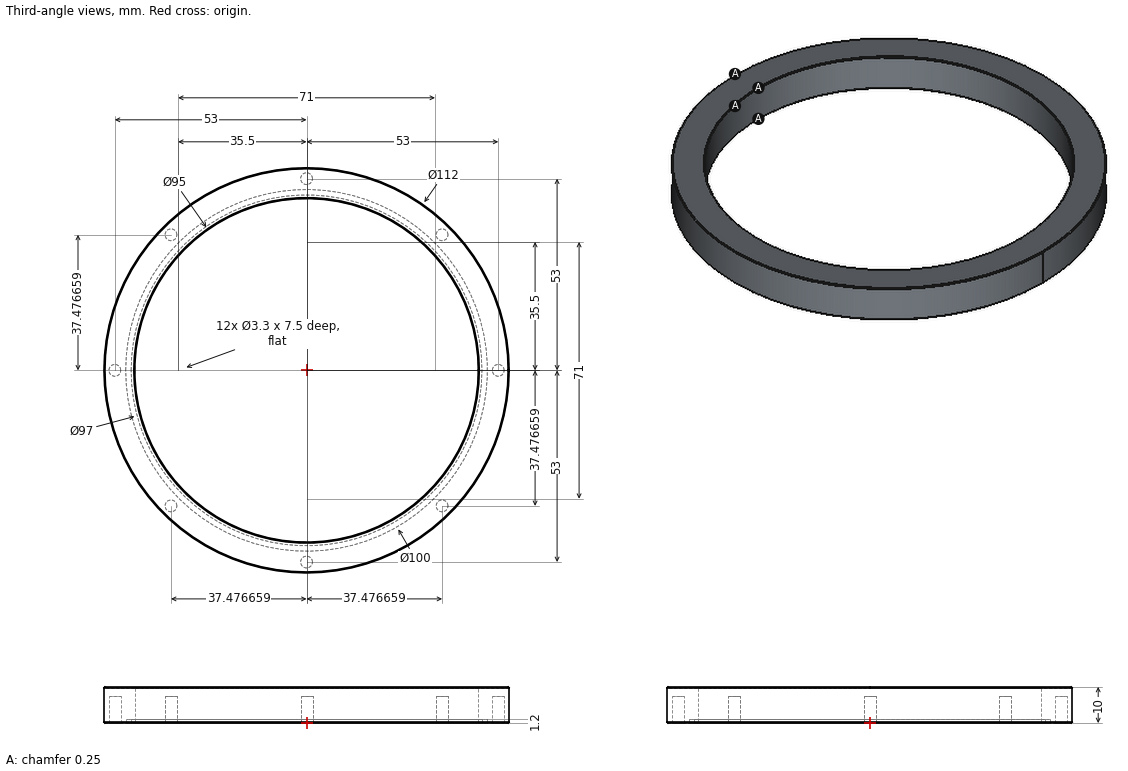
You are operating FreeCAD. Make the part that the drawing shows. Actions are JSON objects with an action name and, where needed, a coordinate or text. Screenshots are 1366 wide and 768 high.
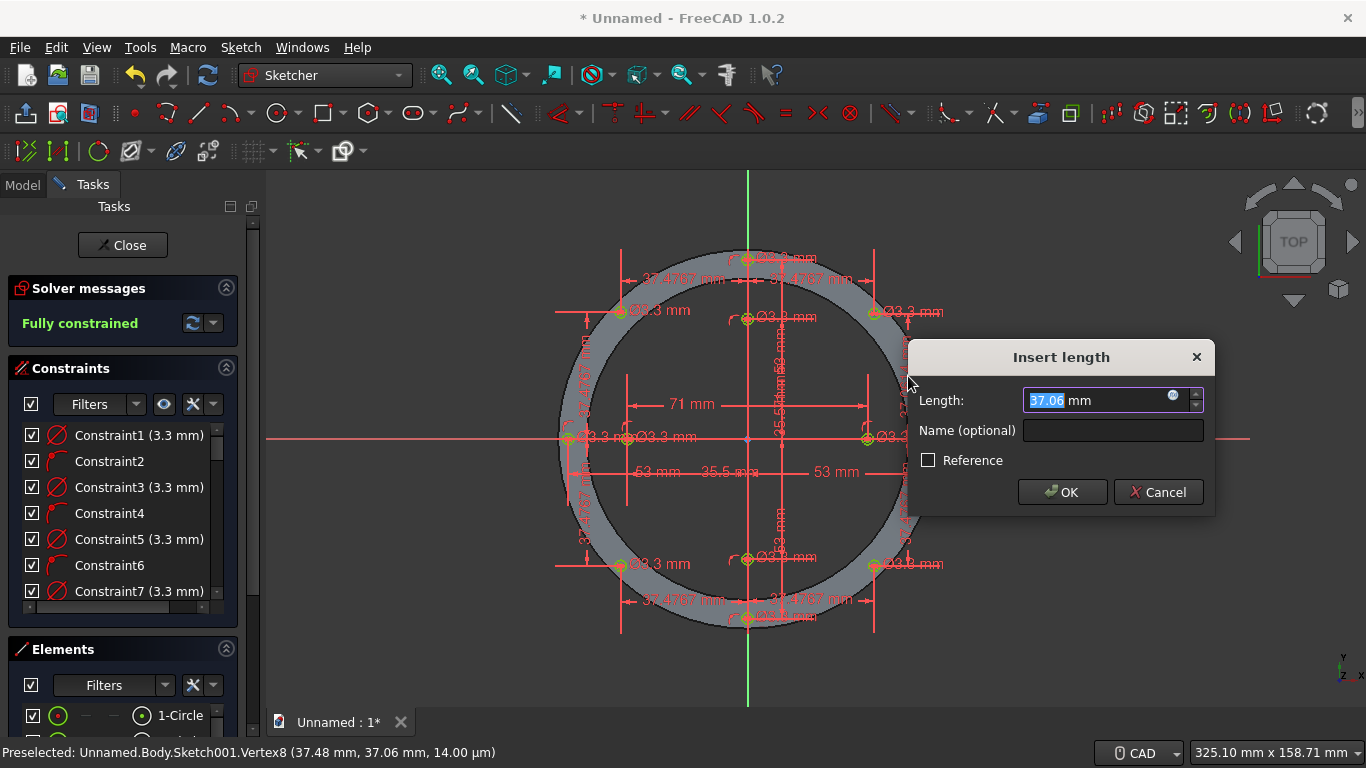
{"action": "type", "text": "37.476659"}
{"action": "key", "text": "Return"}
{"action": "key", "text": "Escape"}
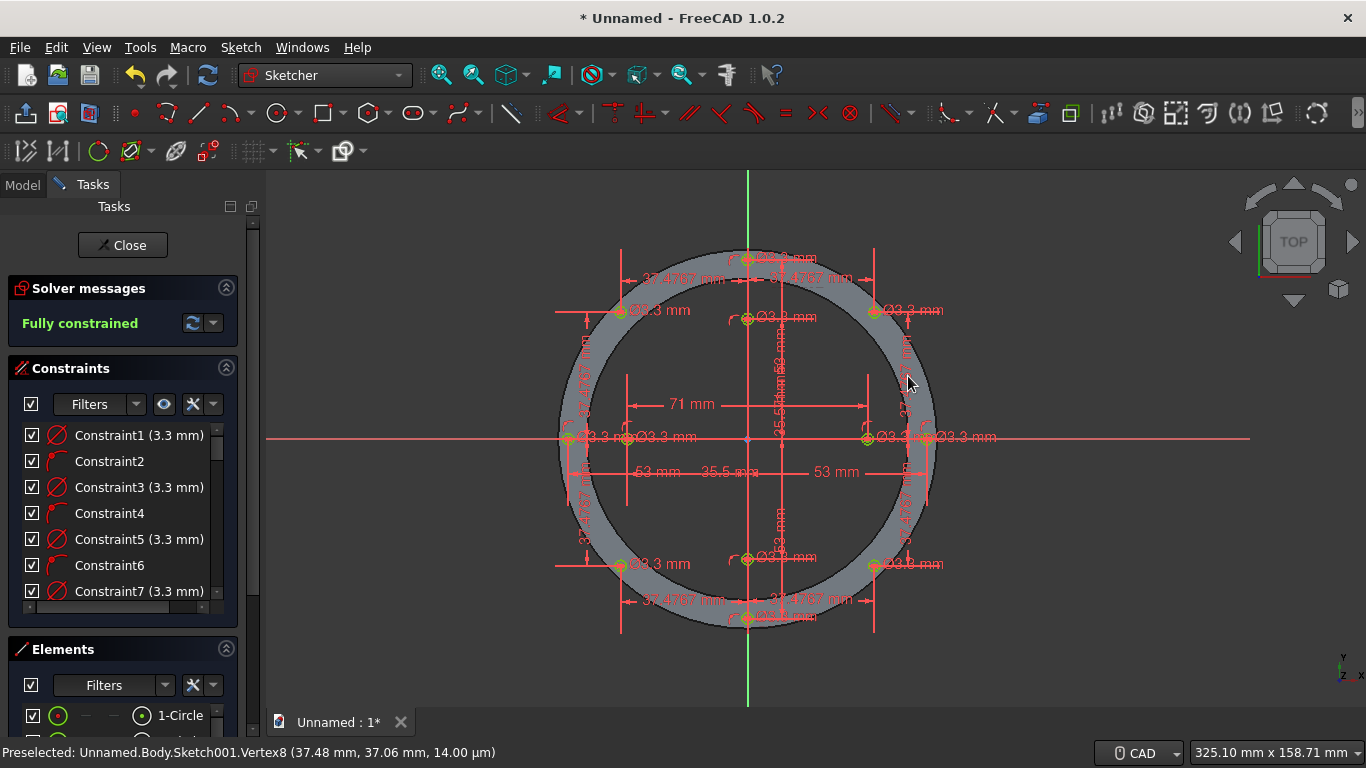
{"action": "left_click", "coordinate": [123, 245]}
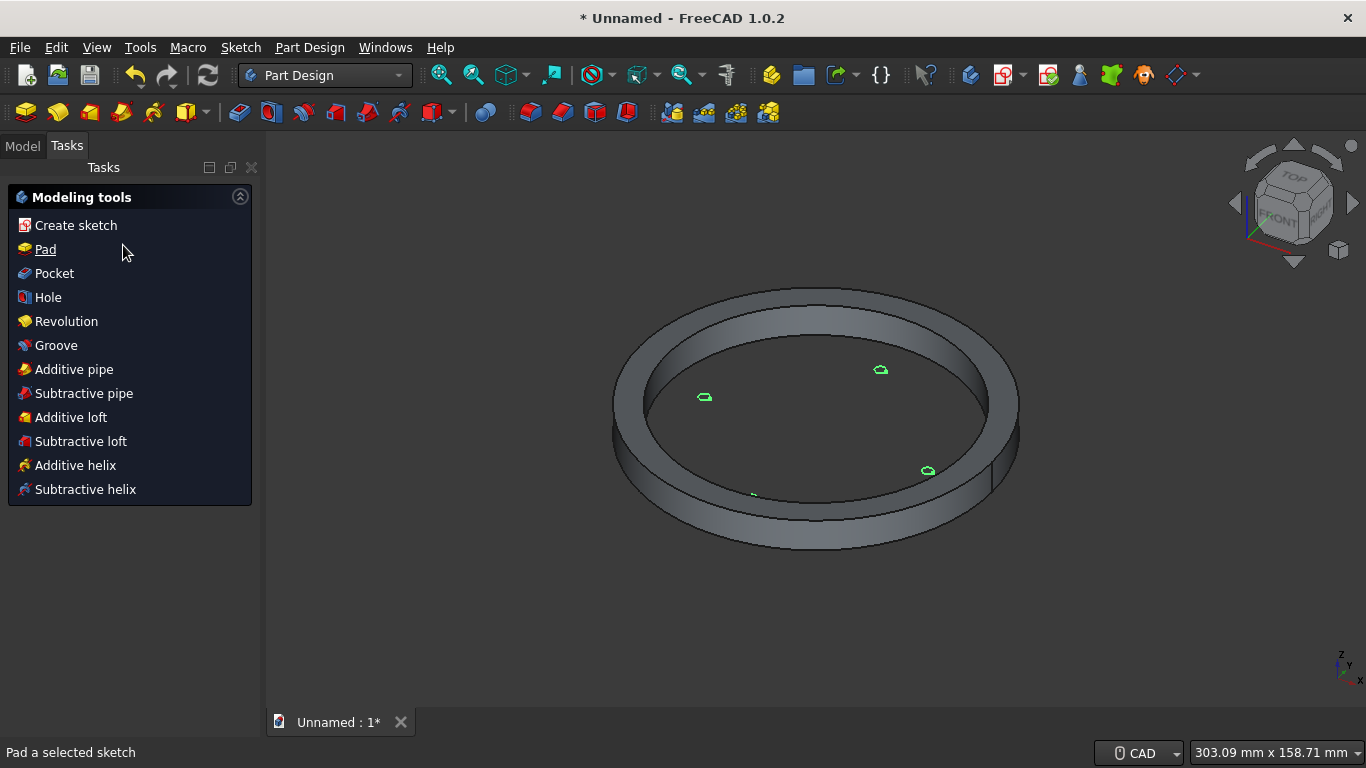
{"action": "left_click", "coordinate": [272, 112]}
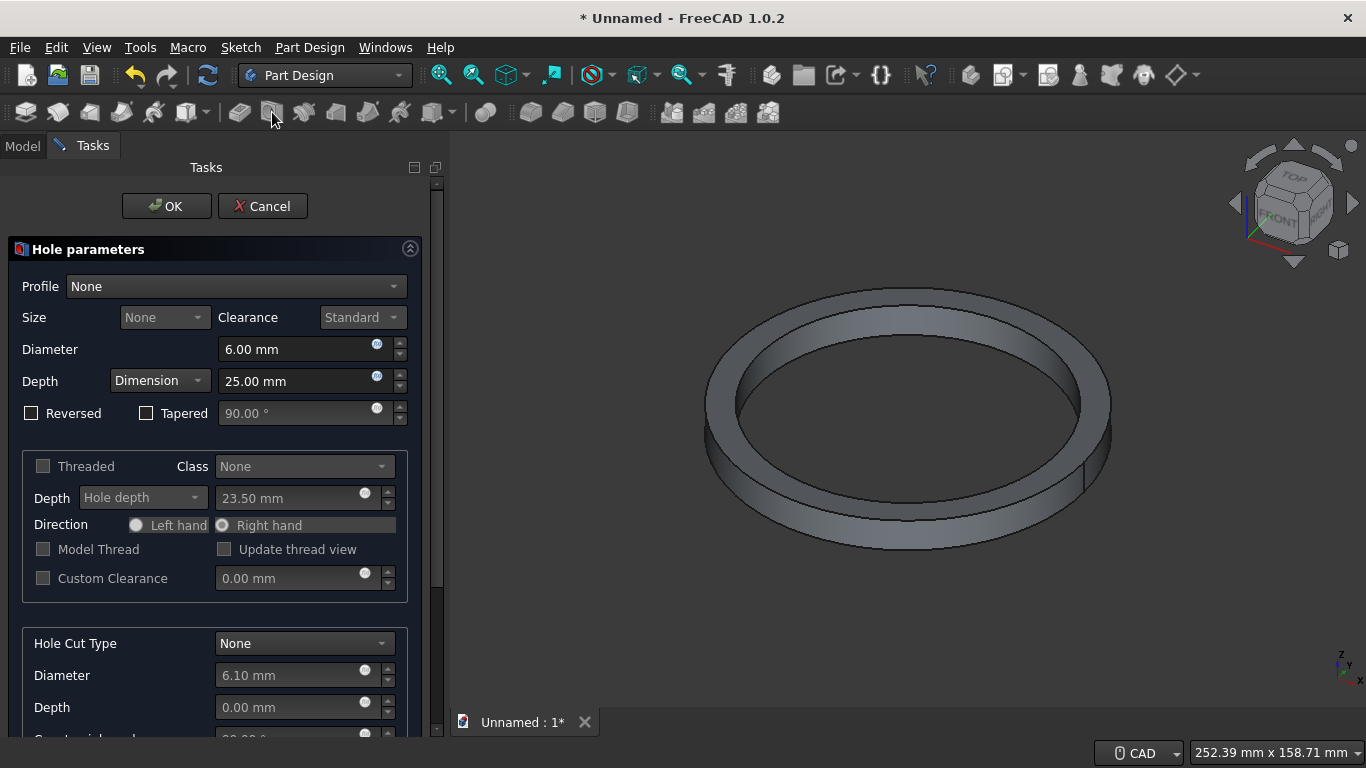
{"action": "triple_click", "coordinate": [305, 349]}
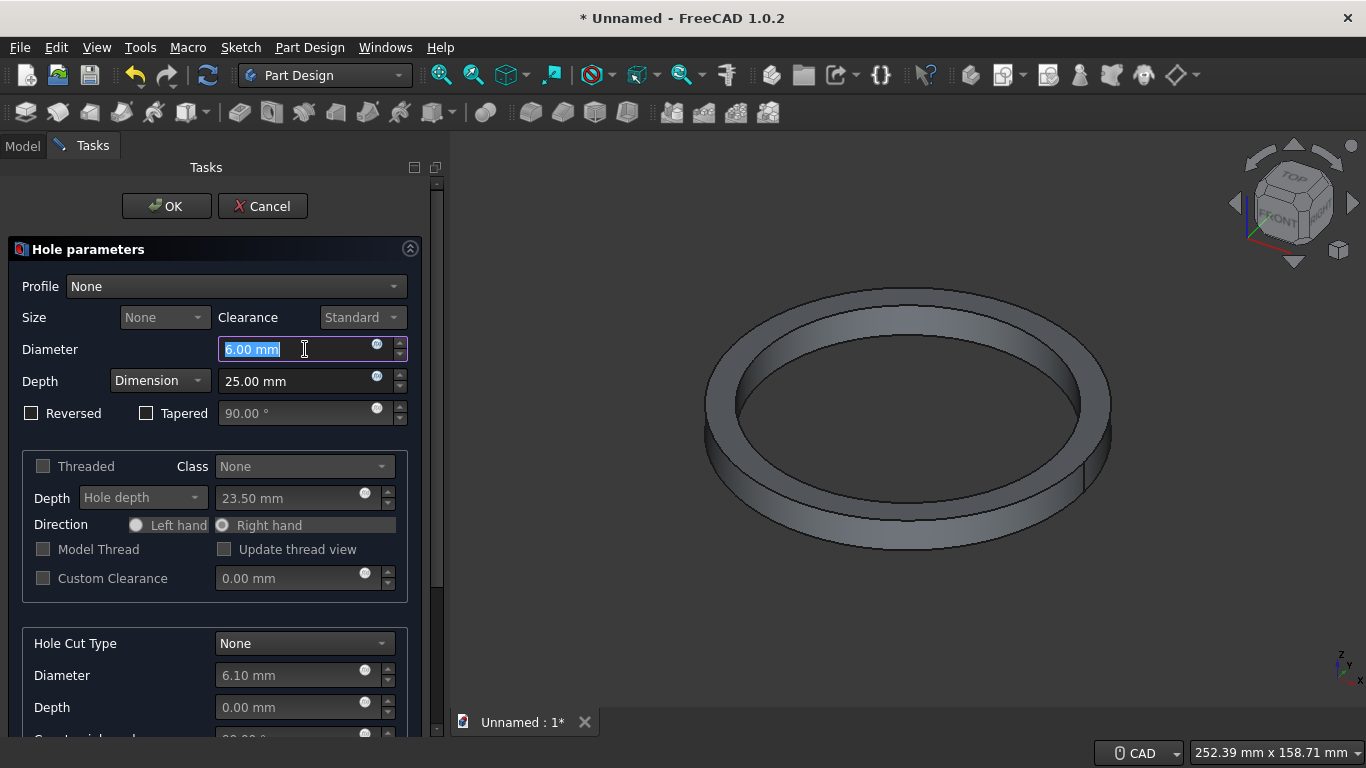
{"action": "type", "text": "3.3"}
{"action": "key", "text": "Tab"}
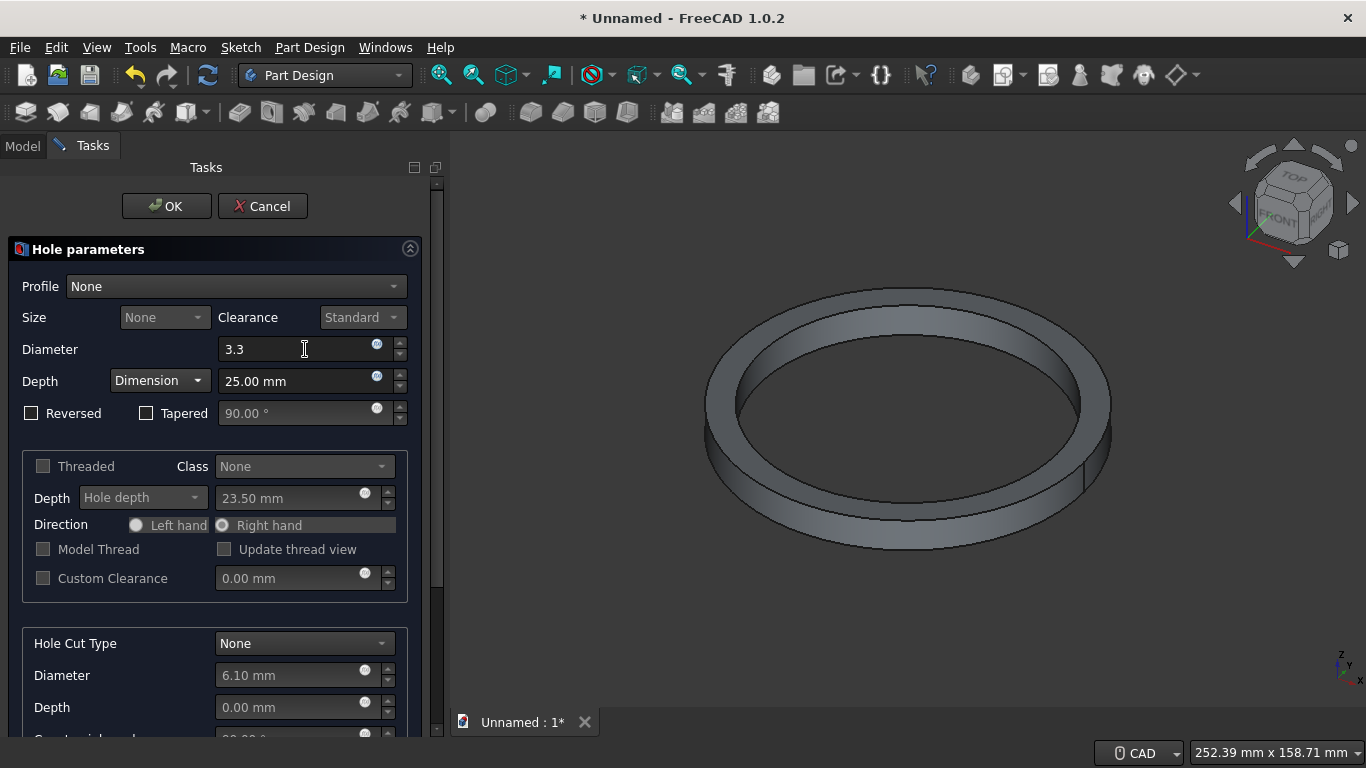
{"action": "triple_click", "coordinate": [305, 381]}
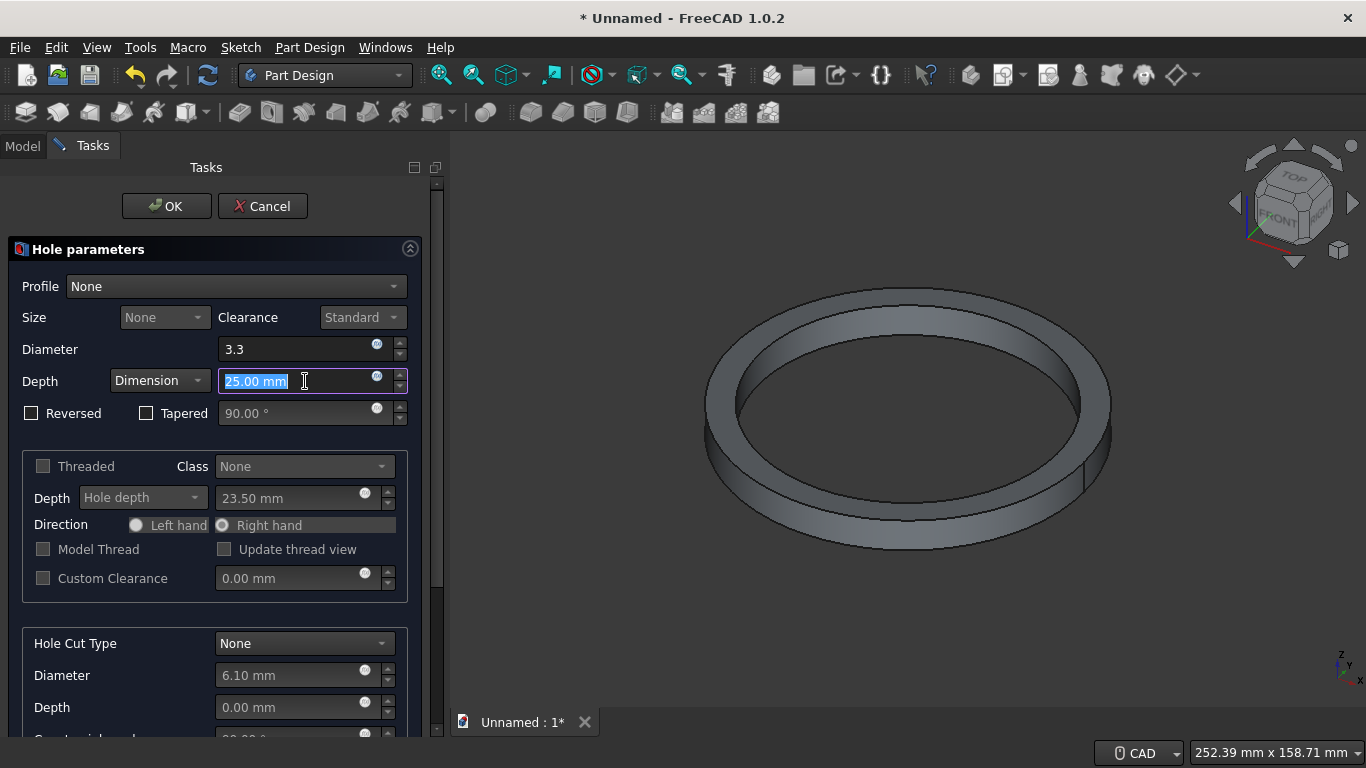
{"action": "type", "text": "7.5"}
{"action": "key", "text": "Tab"}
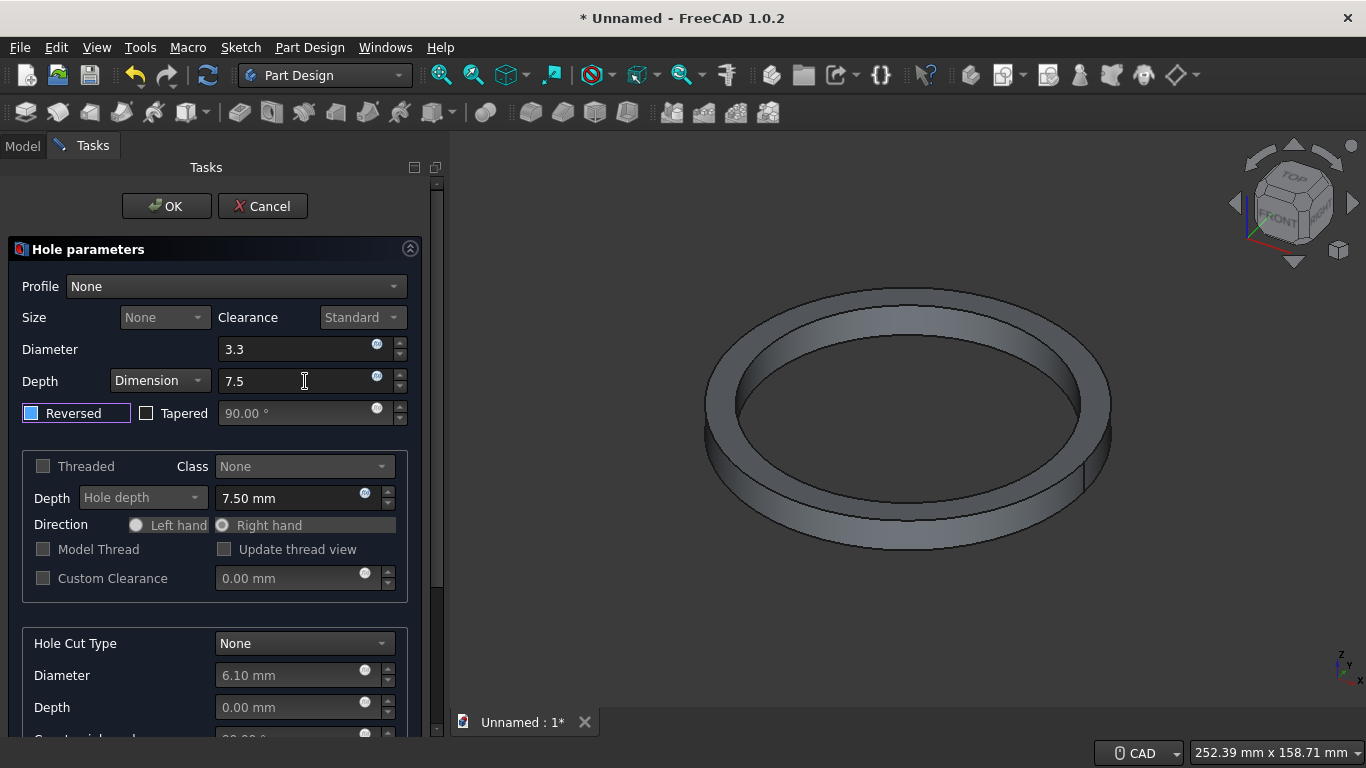
{"action": "left_click", "coordinate": [30, 413]}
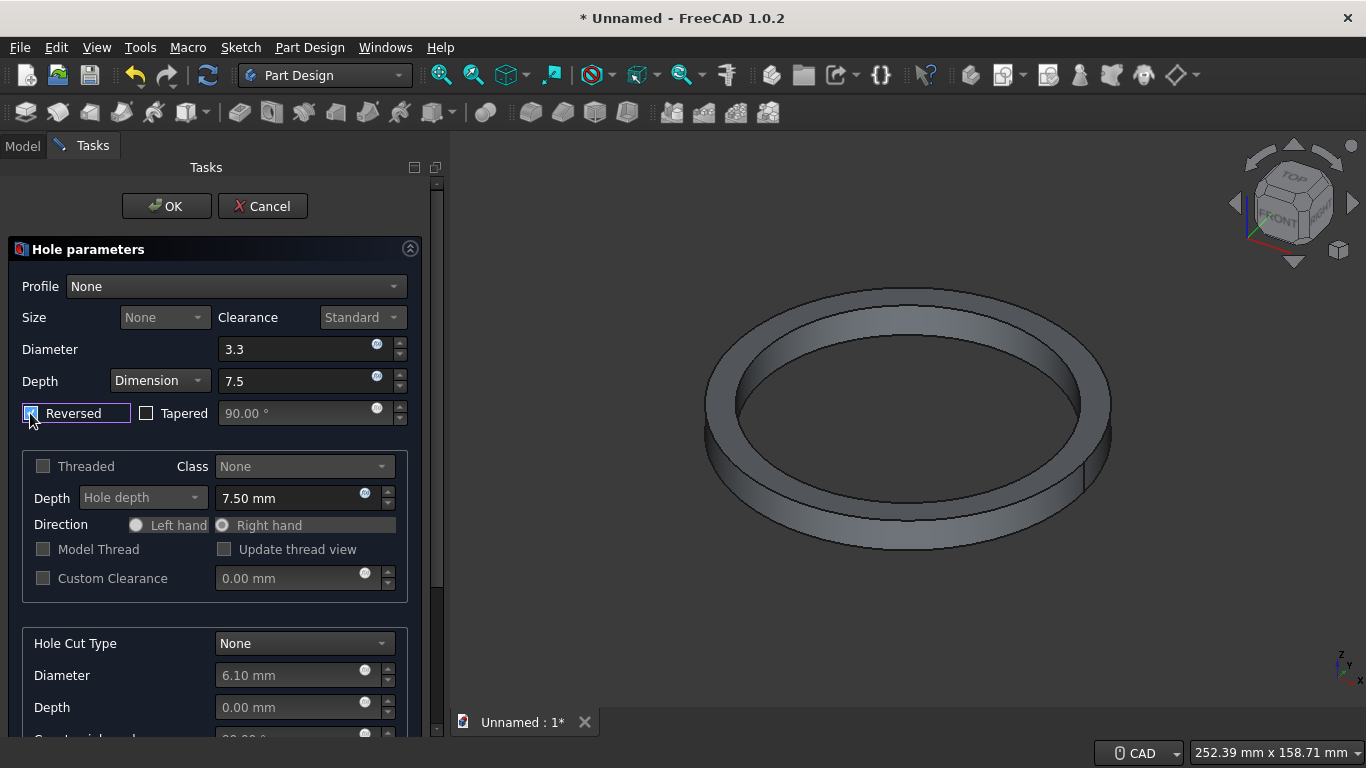
{"action": "scroll", "coordinate": [437, 456], "scroll_direction": "down", "scroll_amount": 3}